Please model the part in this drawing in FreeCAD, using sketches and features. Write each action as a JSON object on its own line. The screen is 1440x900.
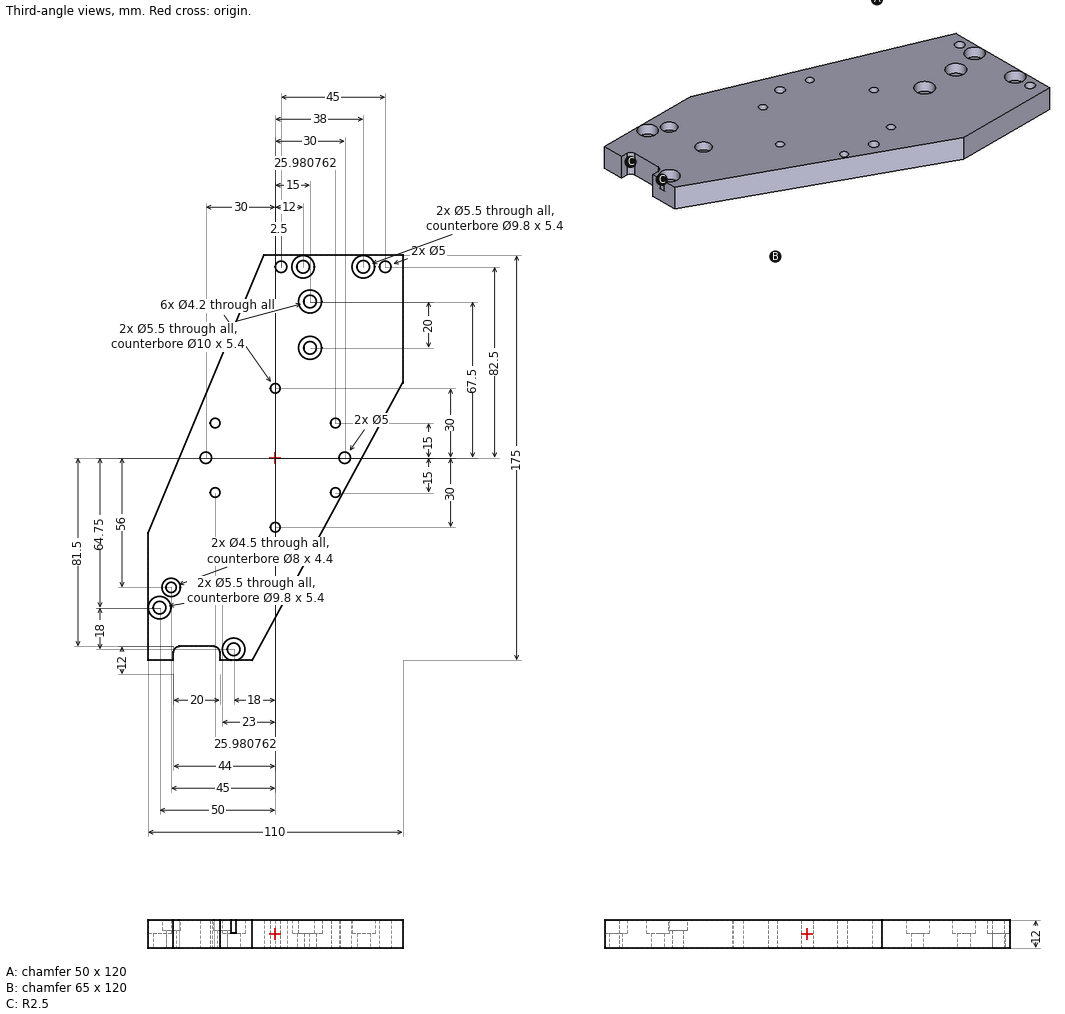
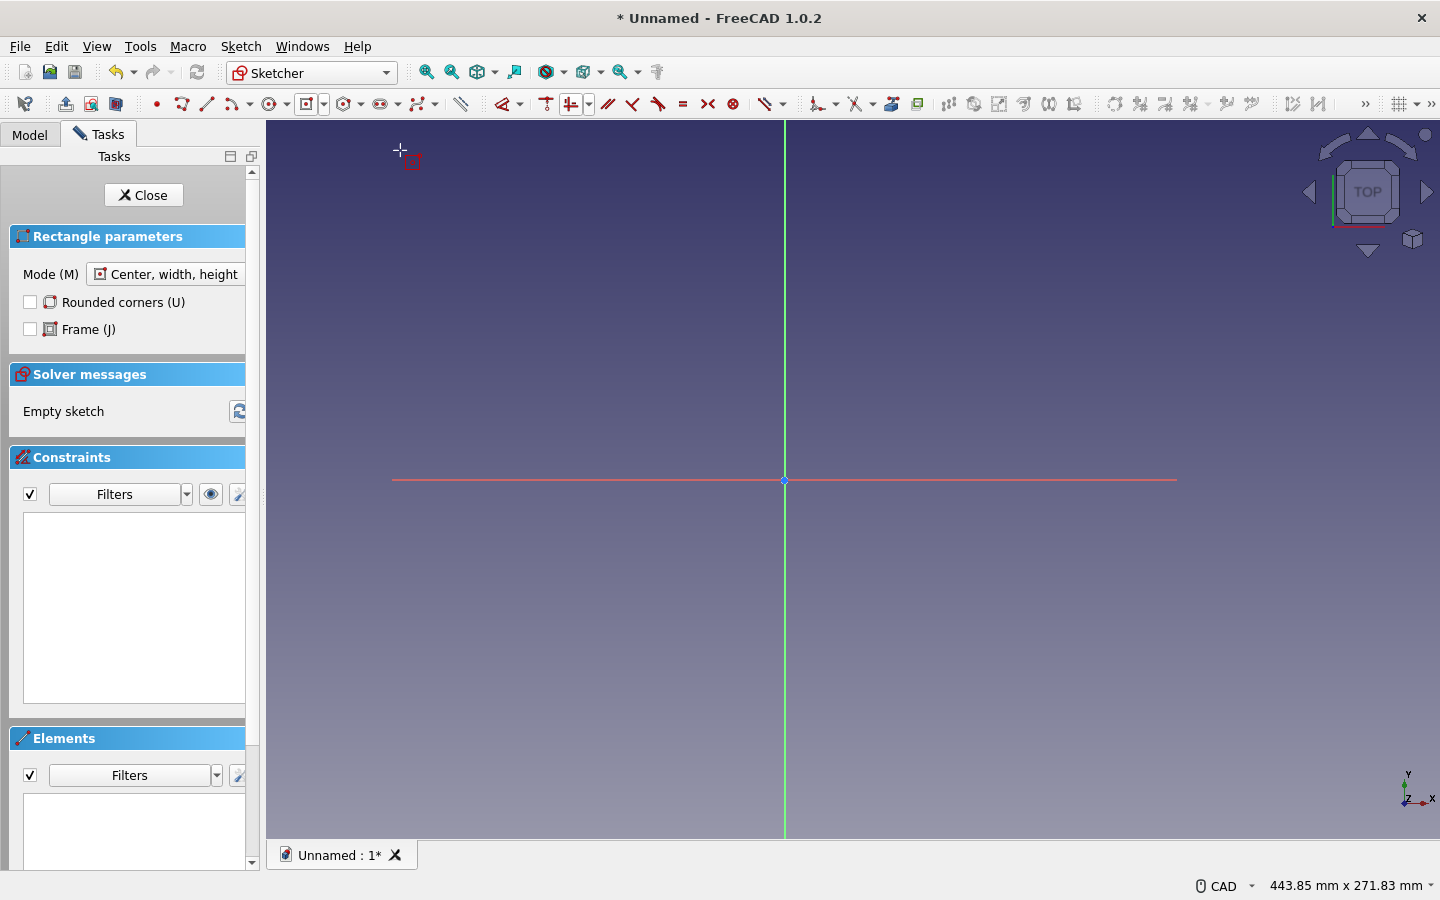
{"action": "left_click", "coordinate": [785, 480]}
{"action": "left_click", "coordinate": [930, 249]}
{"action": "key", "text": "Escape"}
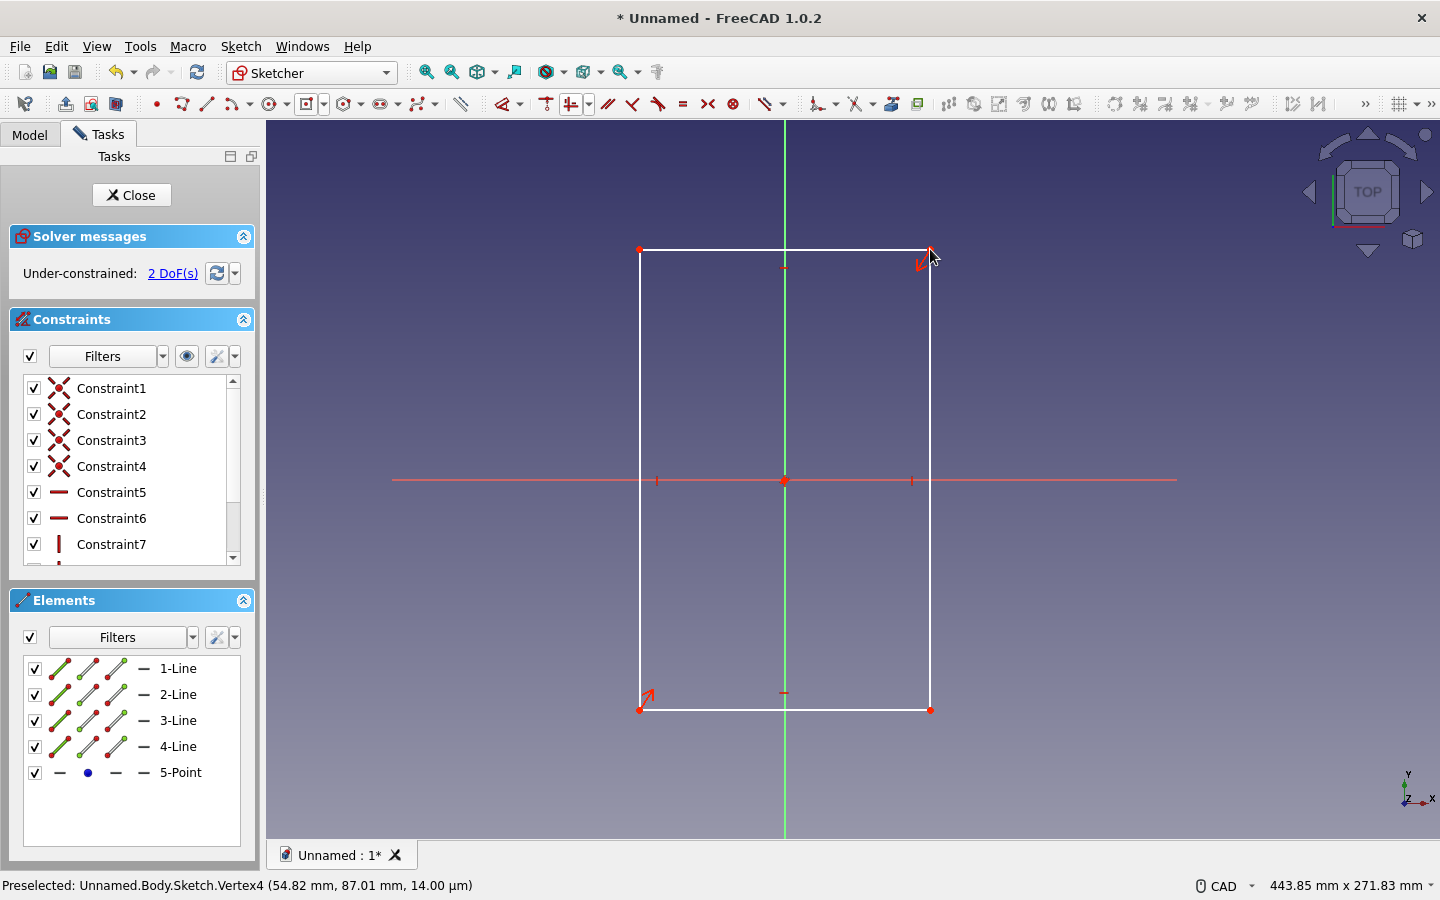
{"action": "left_click", "coordinate": [727, 710]}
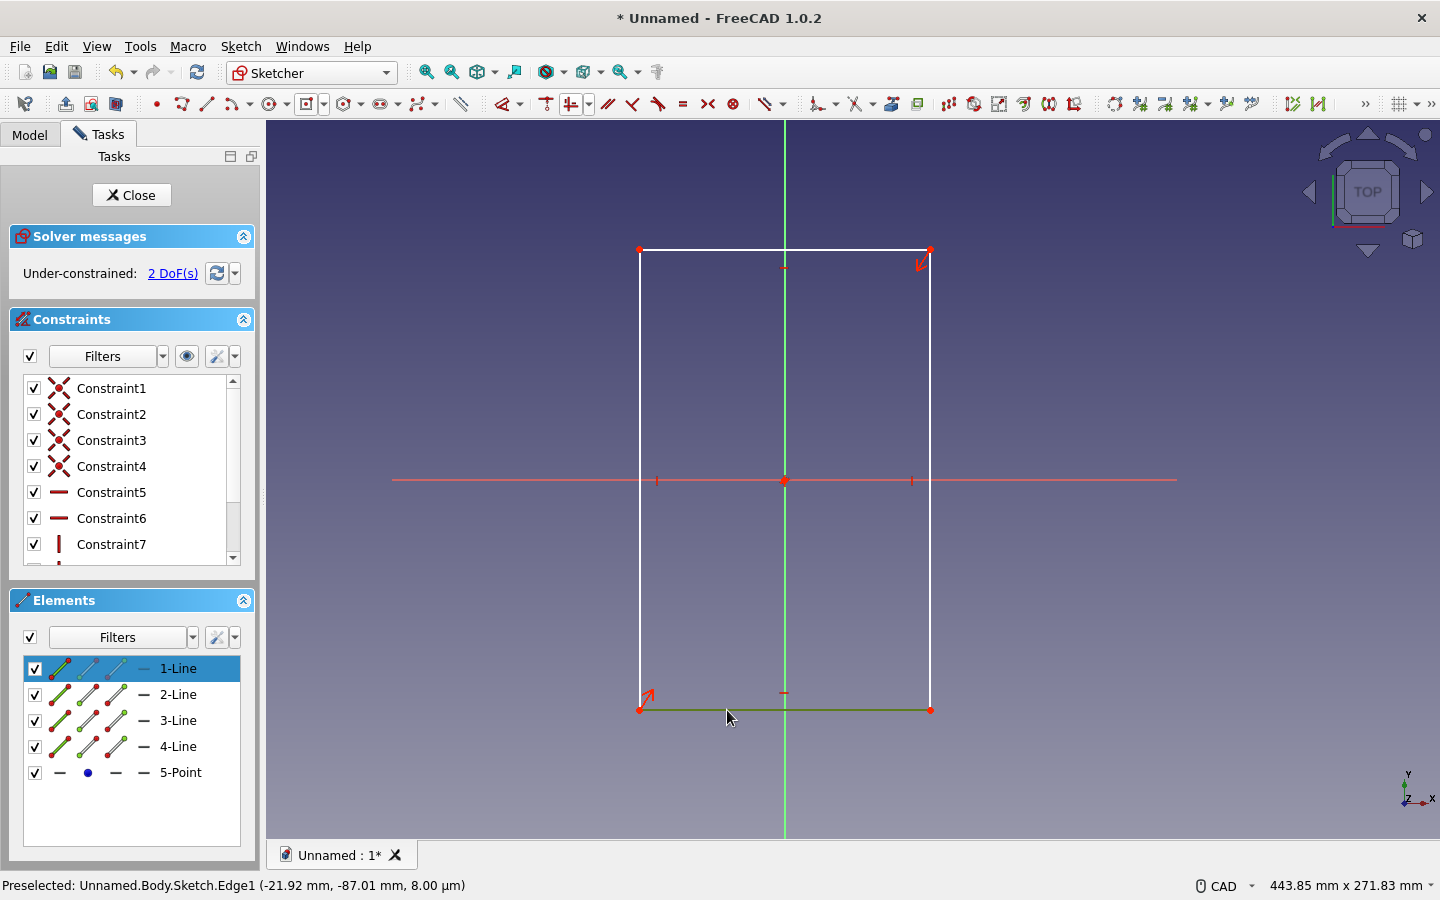
{"action": "key", "text": "l"}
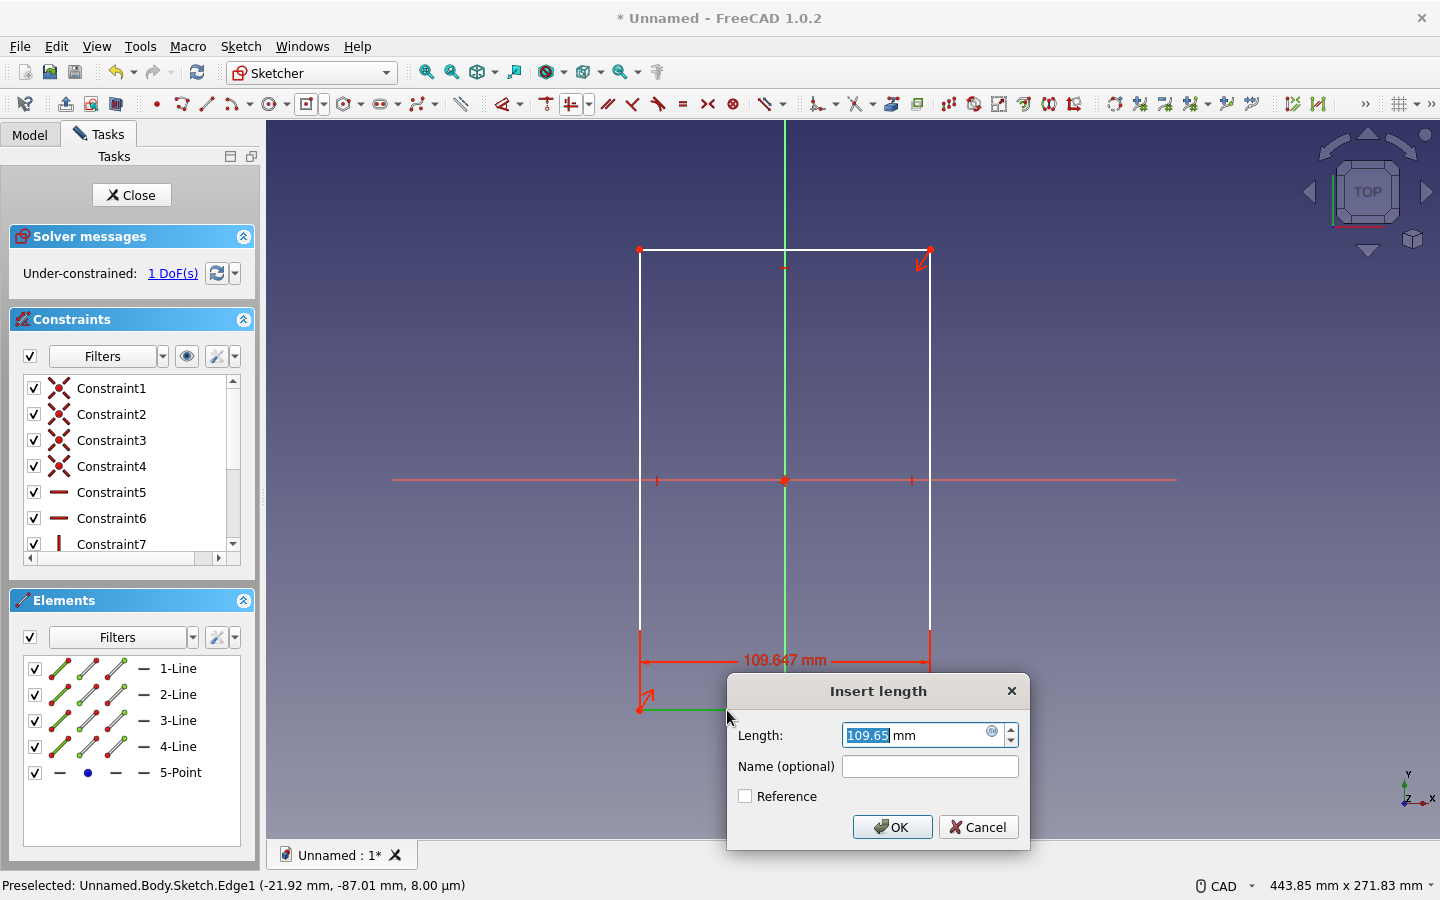
{"action": "type", "text": "110"}
{"action": "key", "text": "Return"}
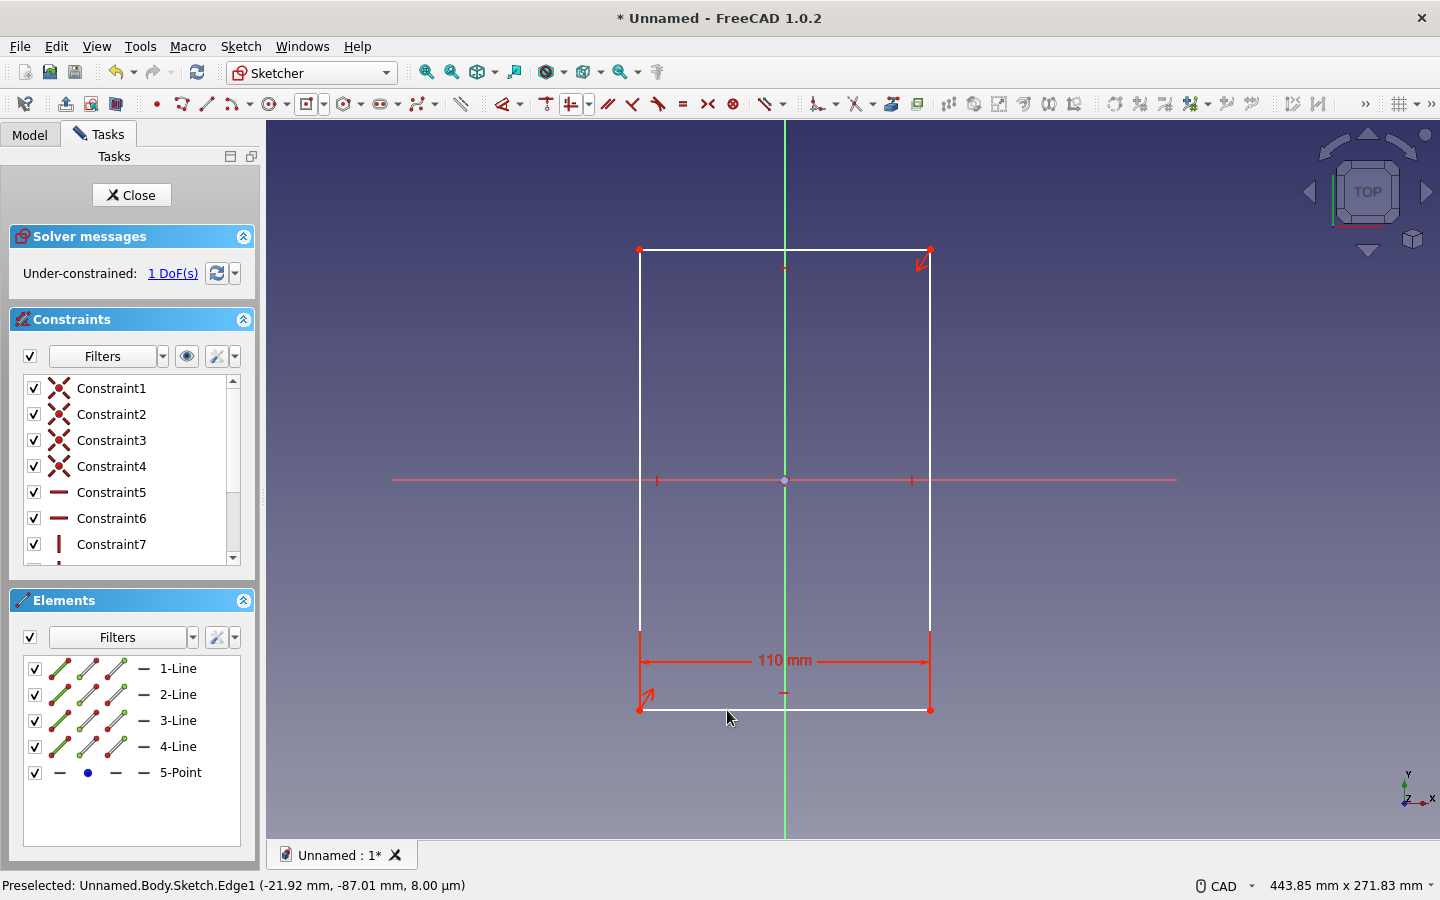
{"action": "left_click", "coordinate": [930, 572]}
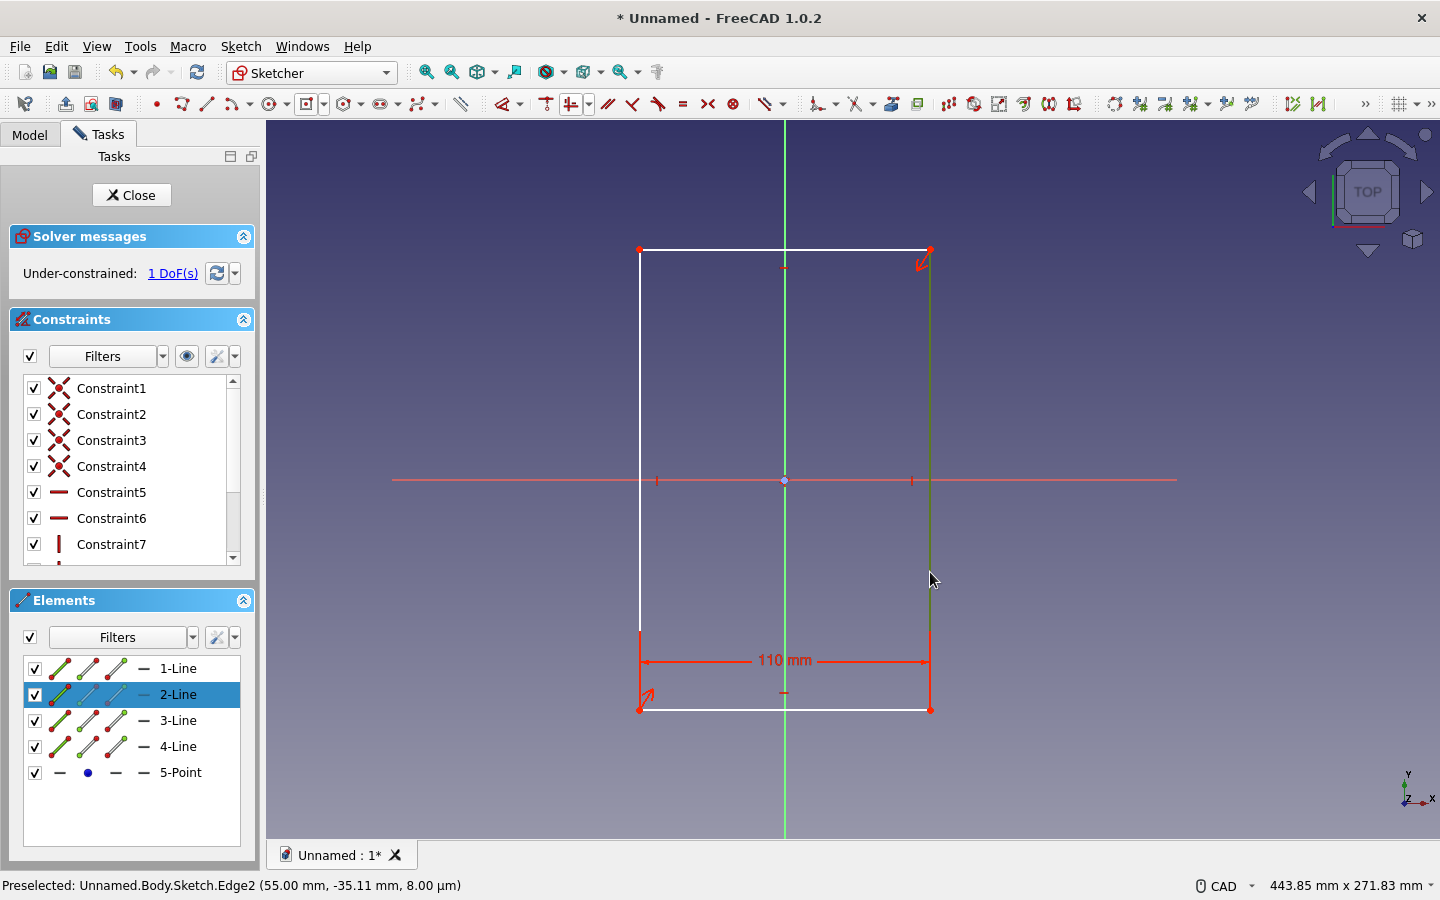
{"action": "key", "text": "i"}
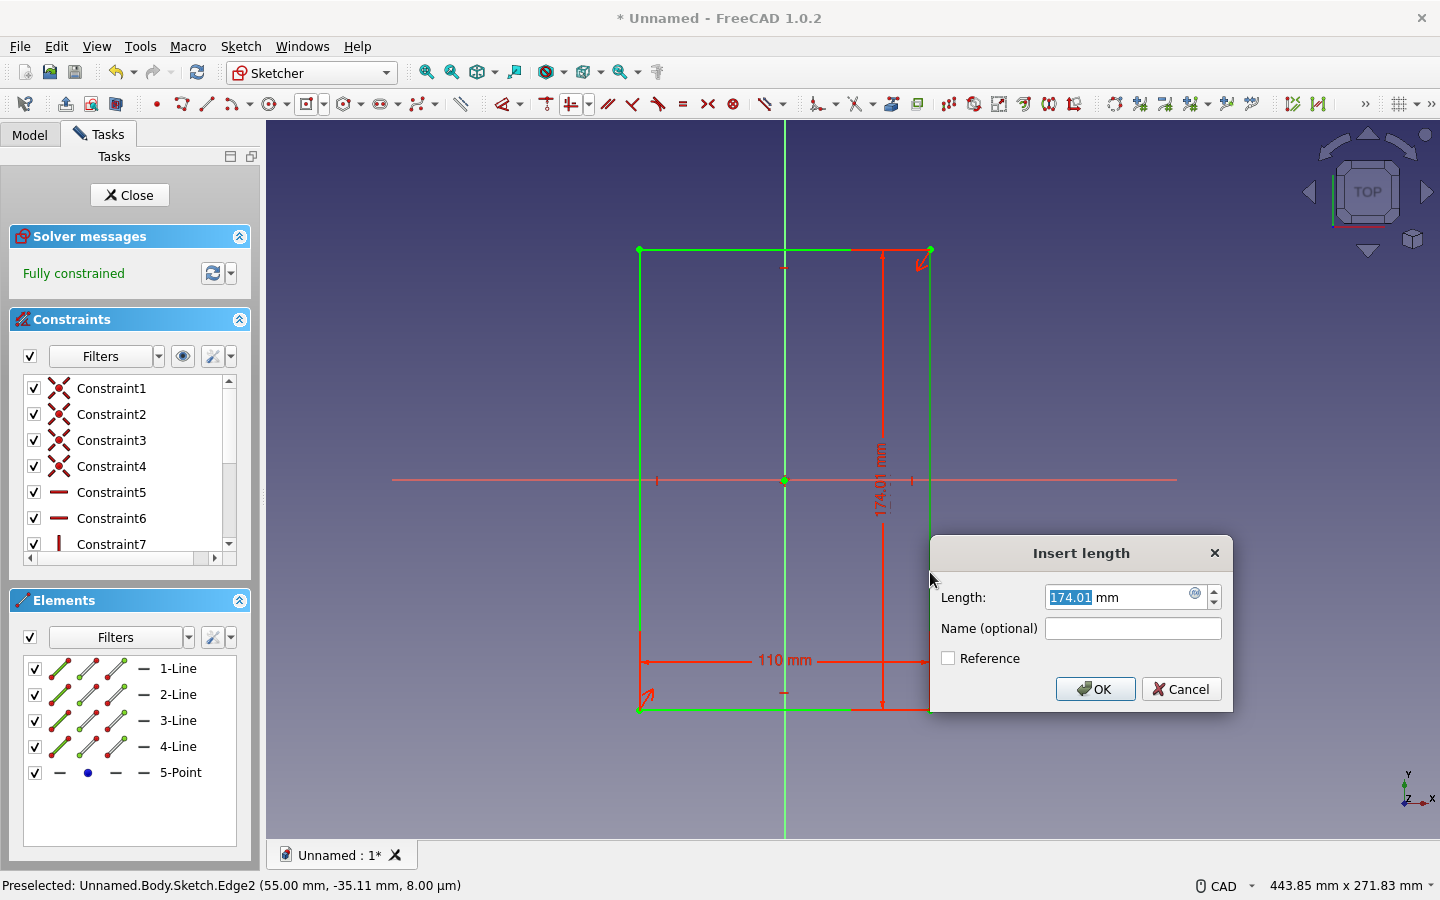
{"action": "type", "text": "175"}
{"action": "key", "text": "Return"}